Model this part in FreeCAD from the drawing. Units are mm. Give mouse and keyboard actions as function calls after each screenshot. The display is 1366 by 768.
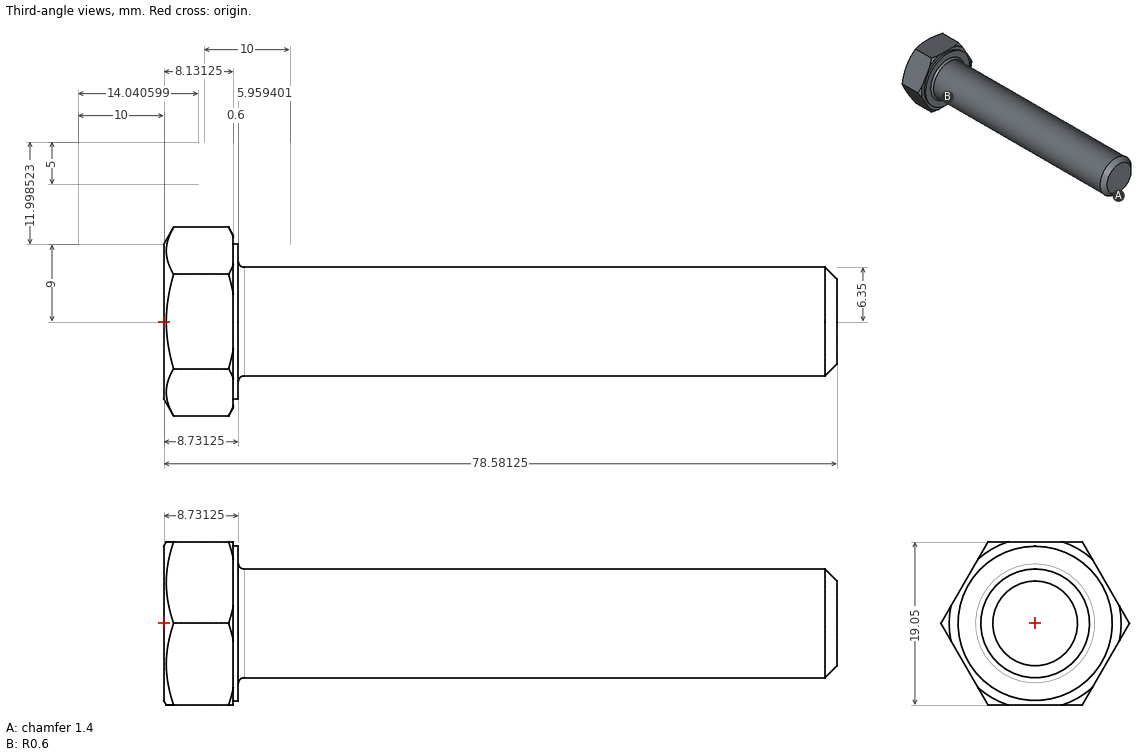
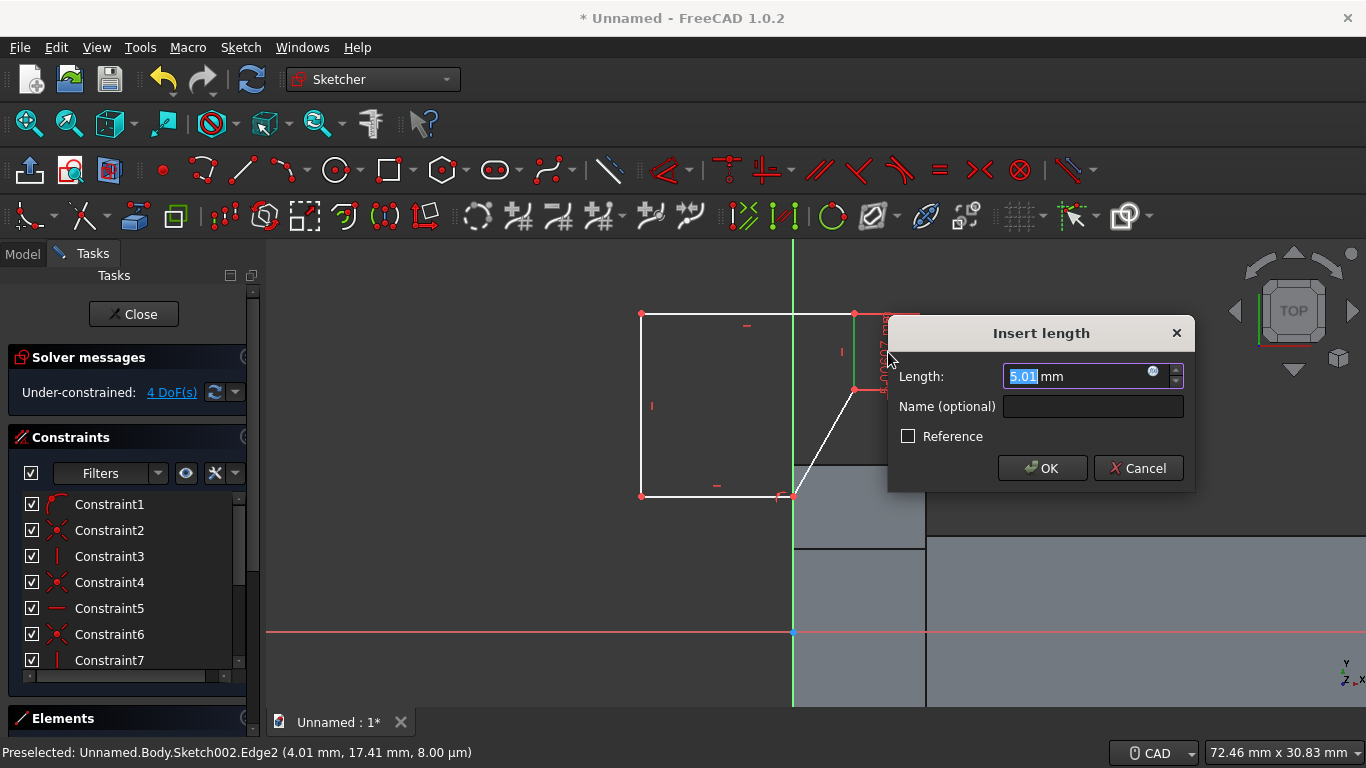
text(5)
key(Return)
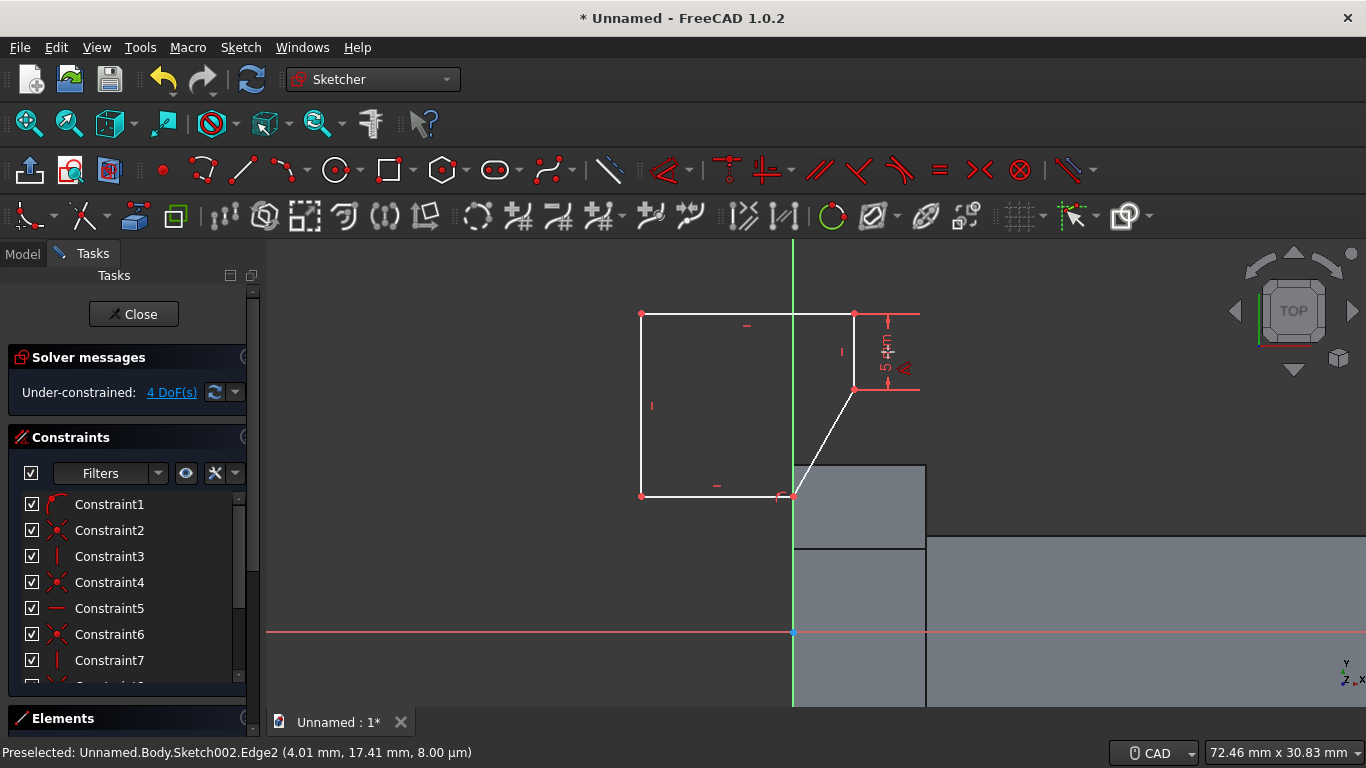
click(687, 497)
click(717, 531)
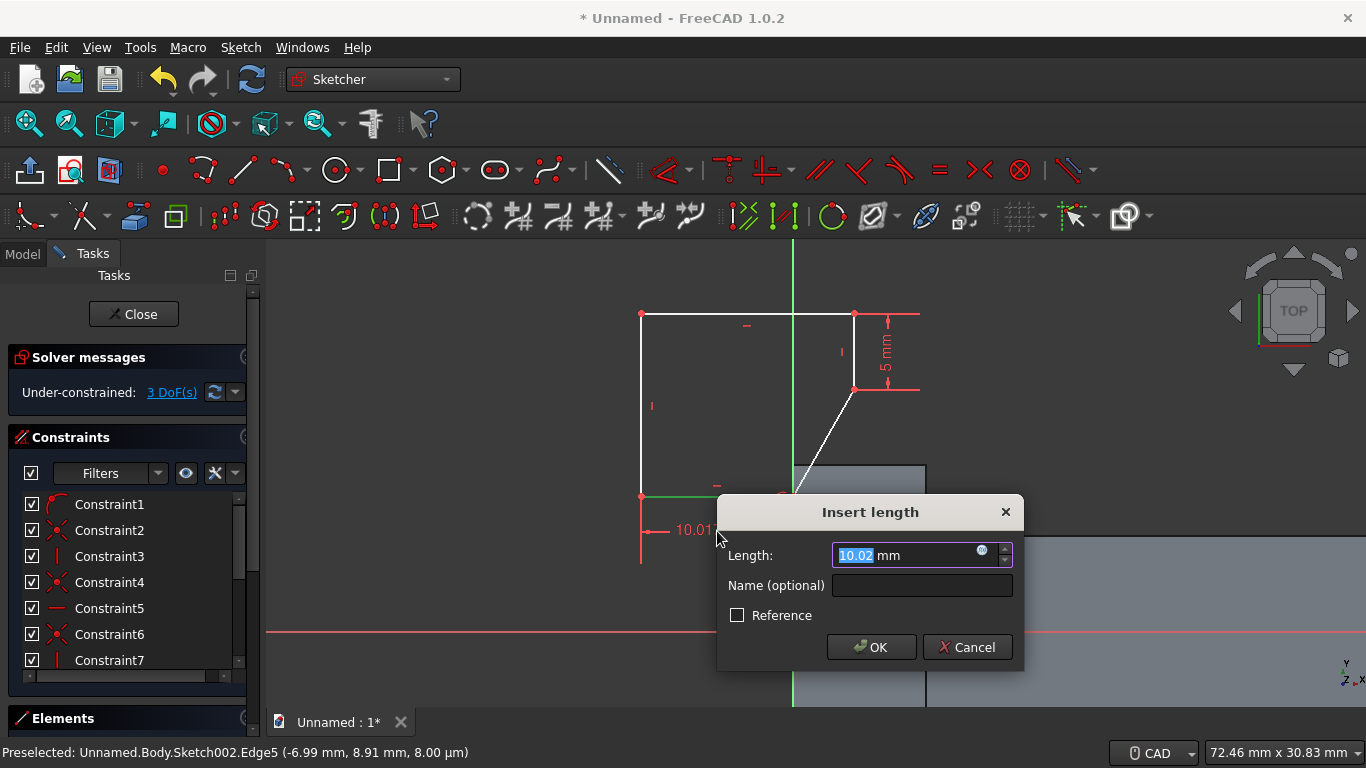
text(10)
key(Return)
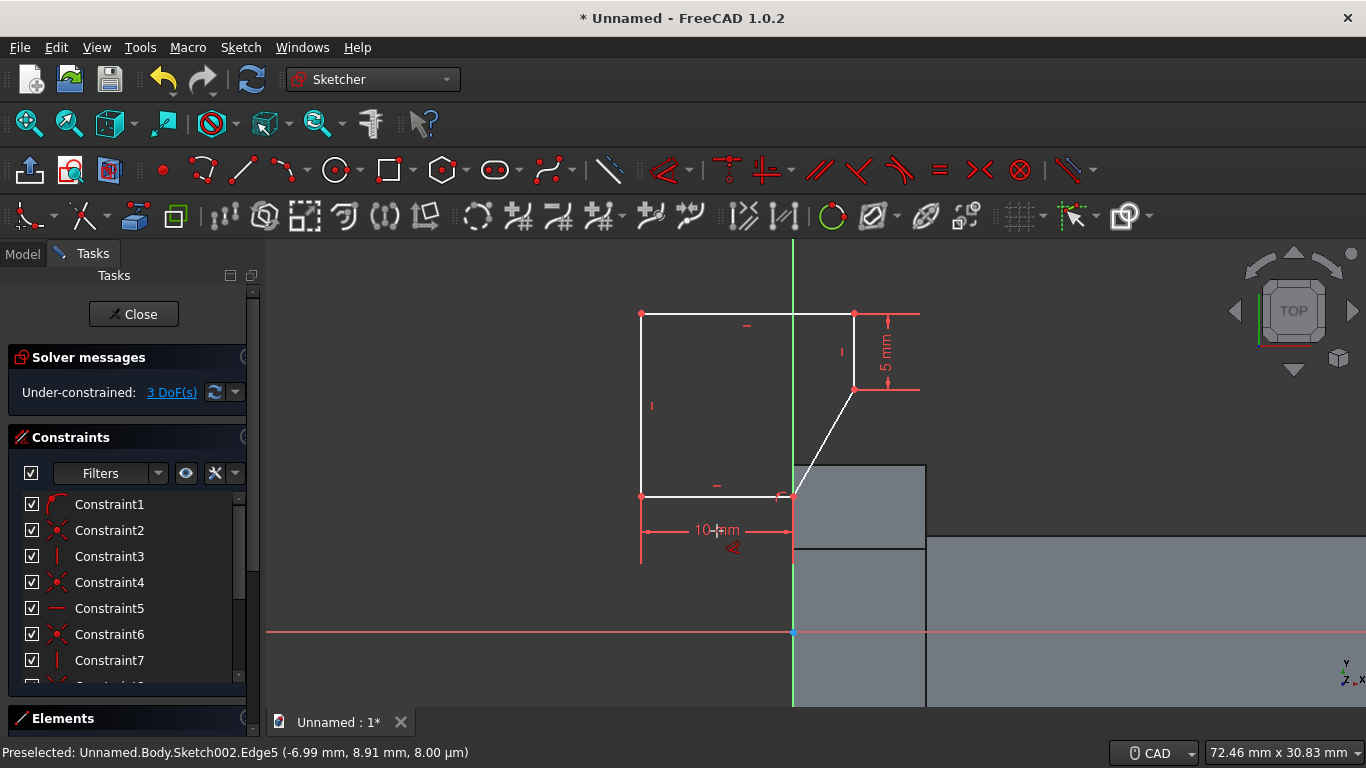
click(793, 497)
click(827, 565)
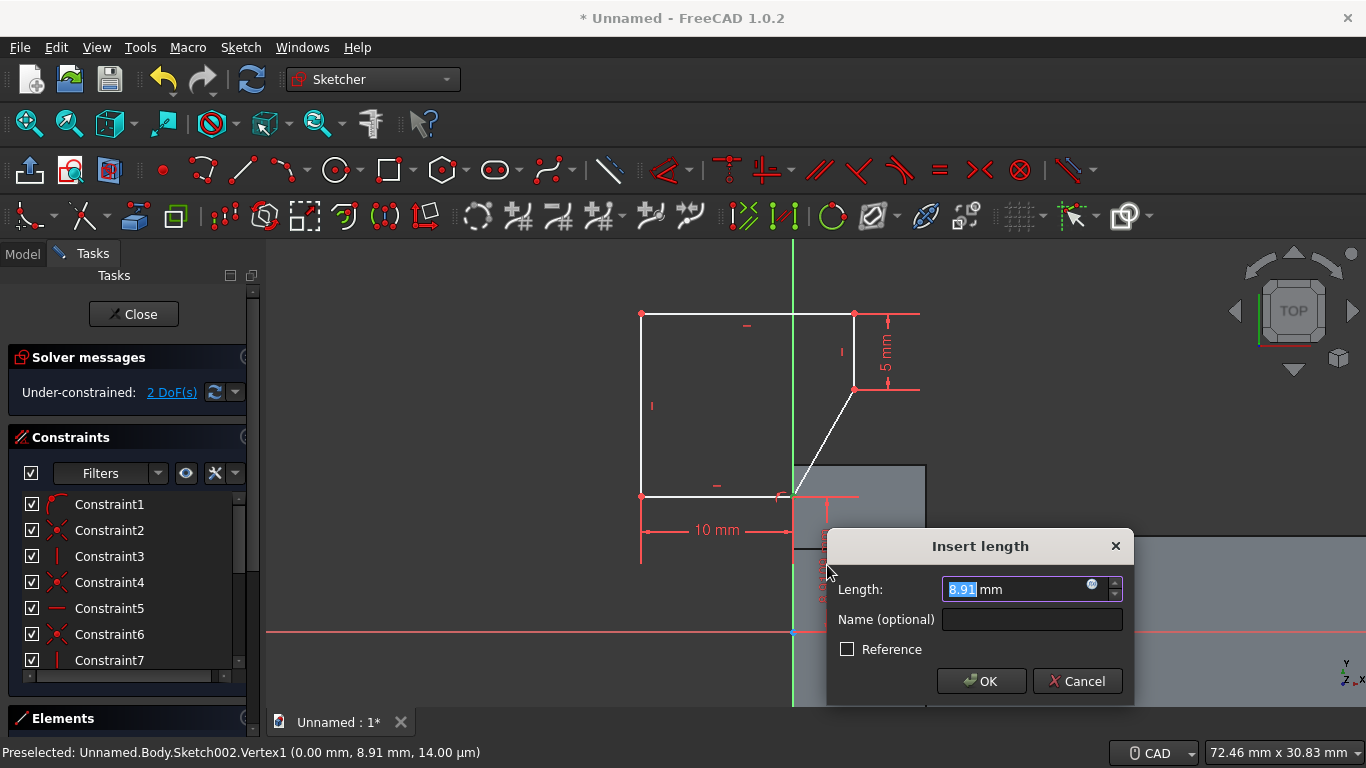
text(9)
key(Return)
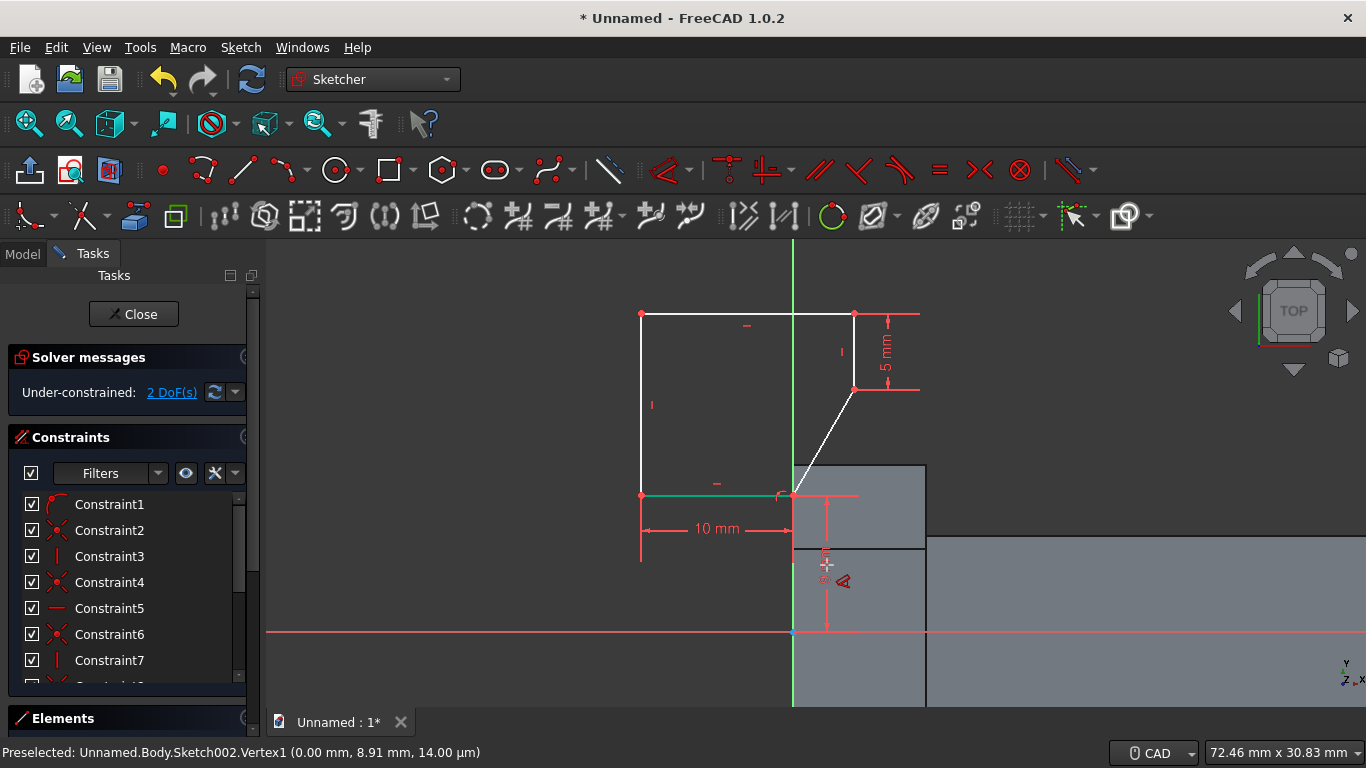
click(790, 314)
click(748, 280)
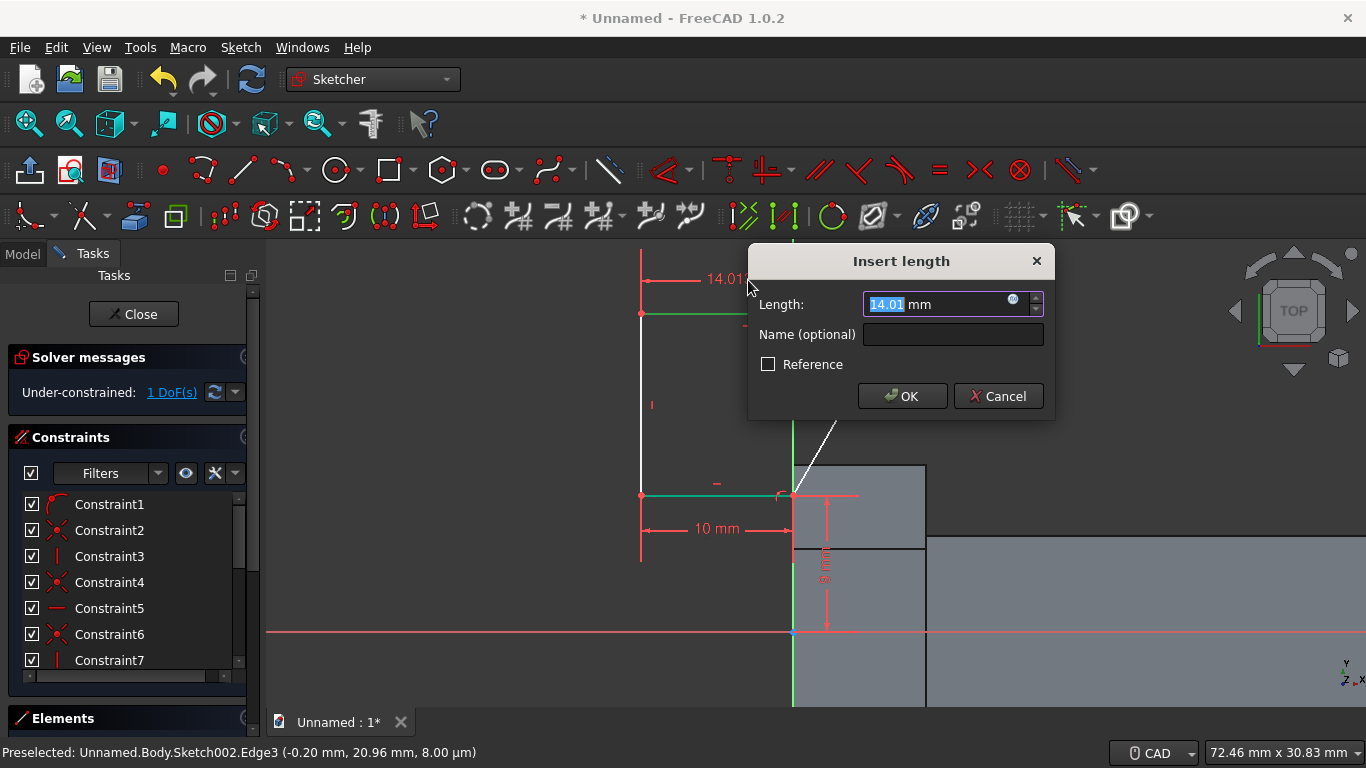
text(14.040599)
key(Return)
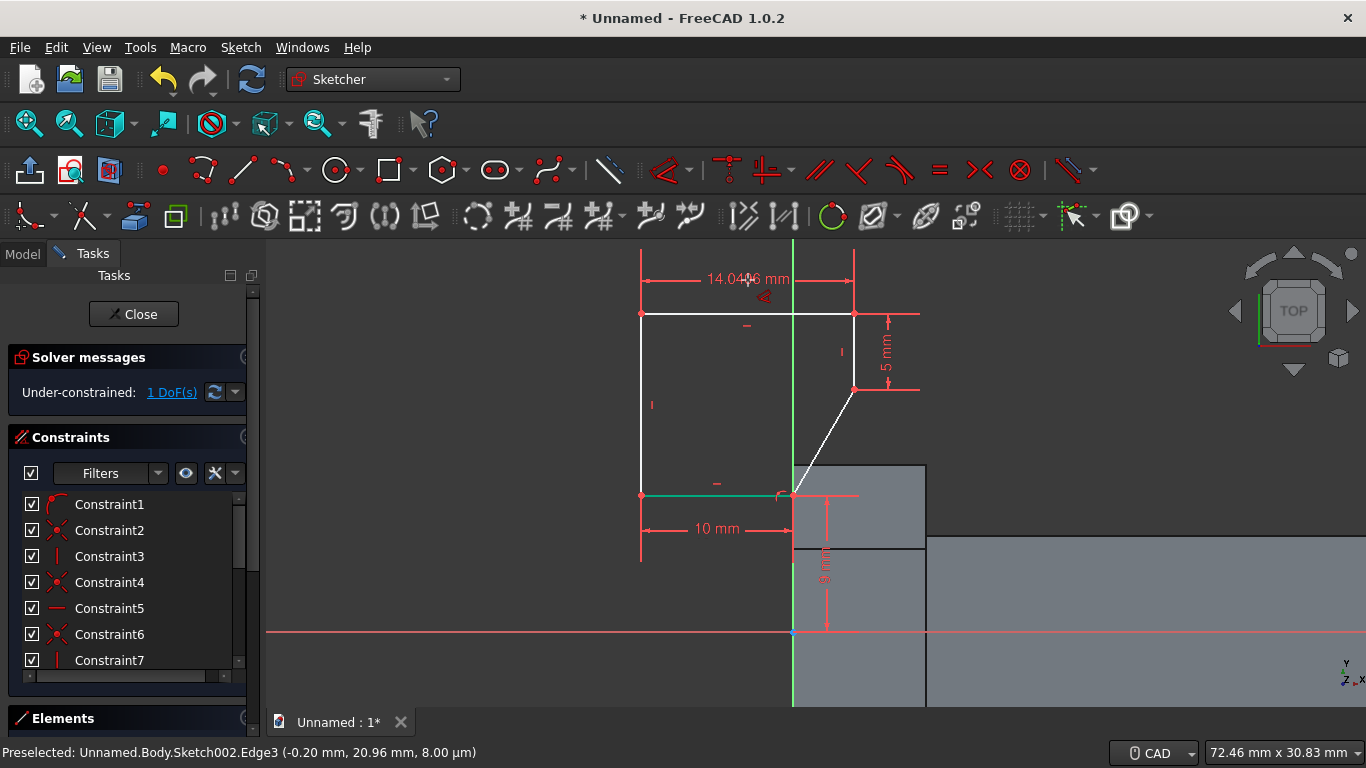
click(641, 368)
click(607, 405)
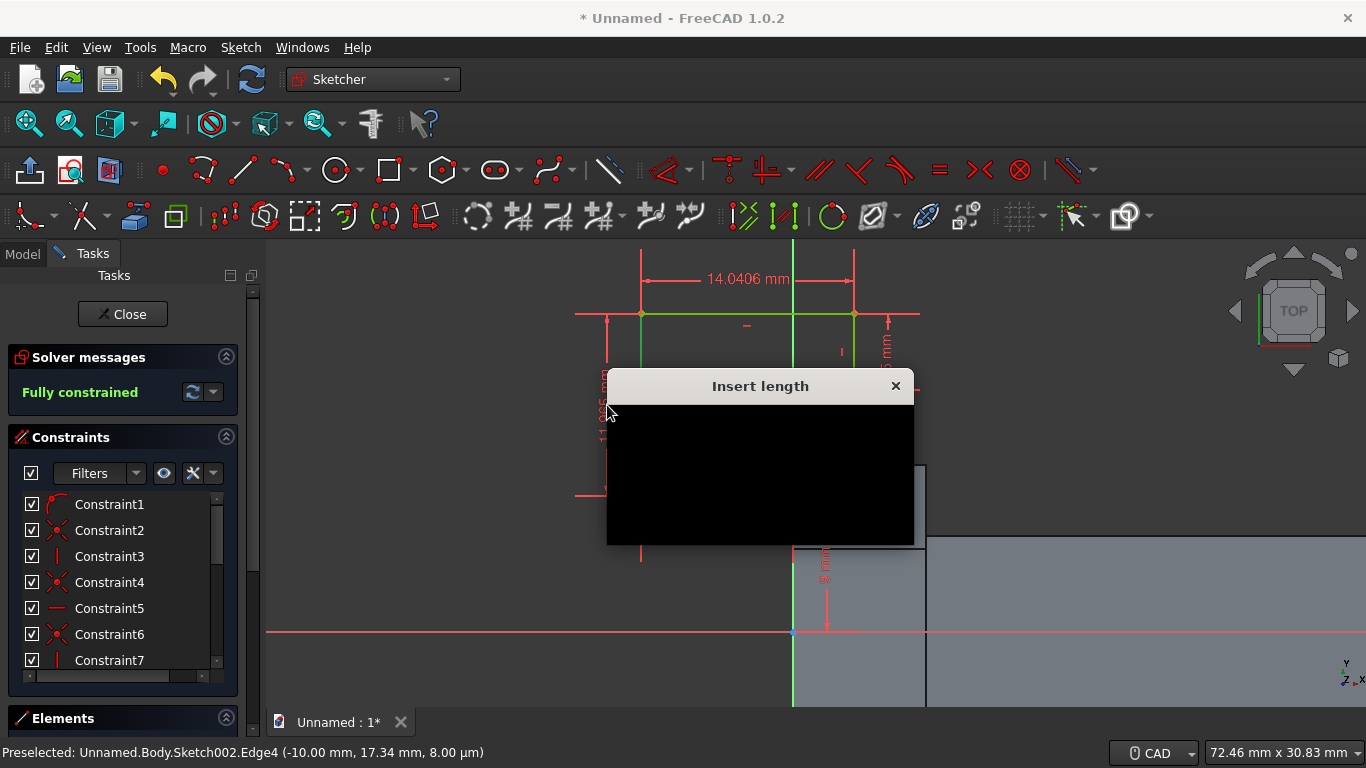
text(11.998523)
key(Return)
key(Escape)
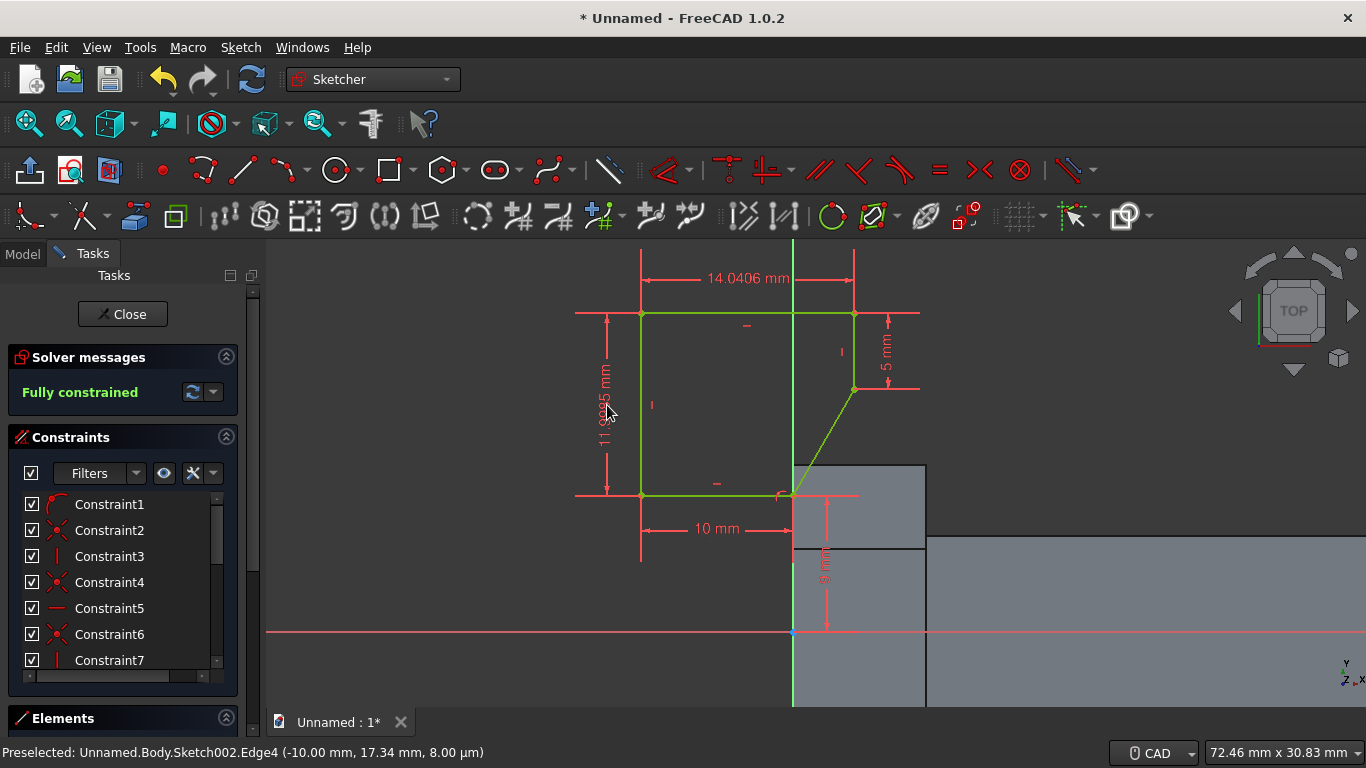
click(123, 314)